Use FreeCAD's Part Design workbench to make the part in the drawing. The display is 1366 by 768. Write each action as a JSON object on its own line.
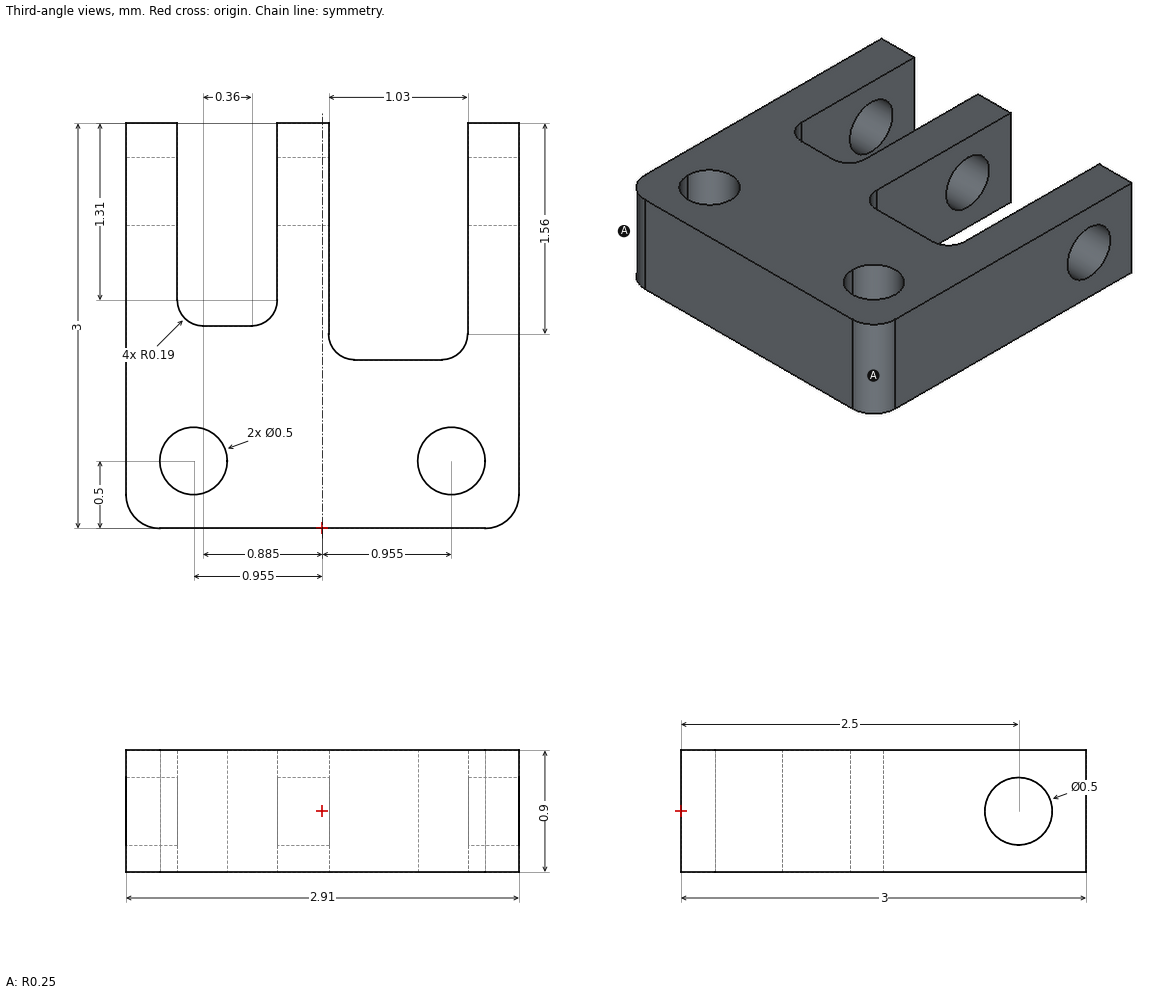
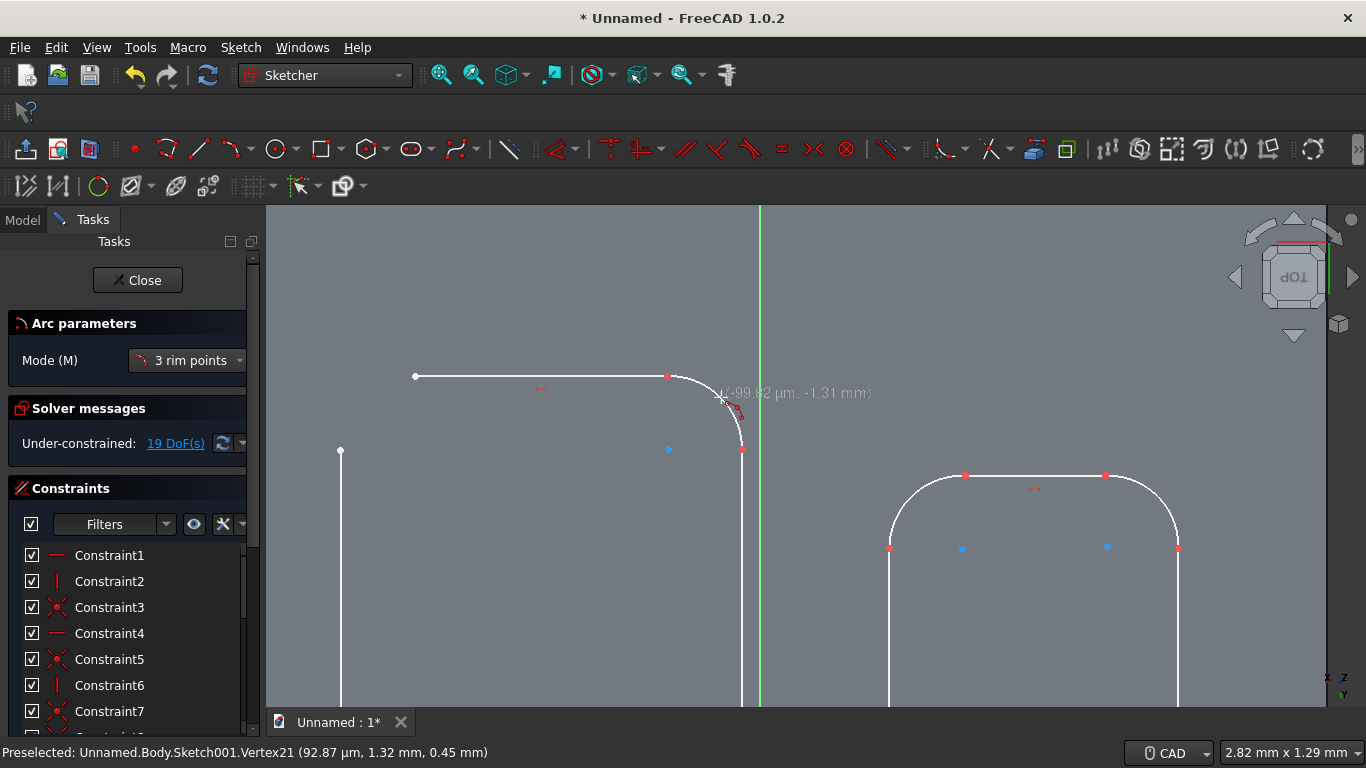
{"action": "left_click", "coordinate": [415, 376]}
{"action": "left_click", "coordinate": [341, 450]}
{"action": "left_click", "coordinate": [363, 397]}
{"action": "key", "text": "Escape"}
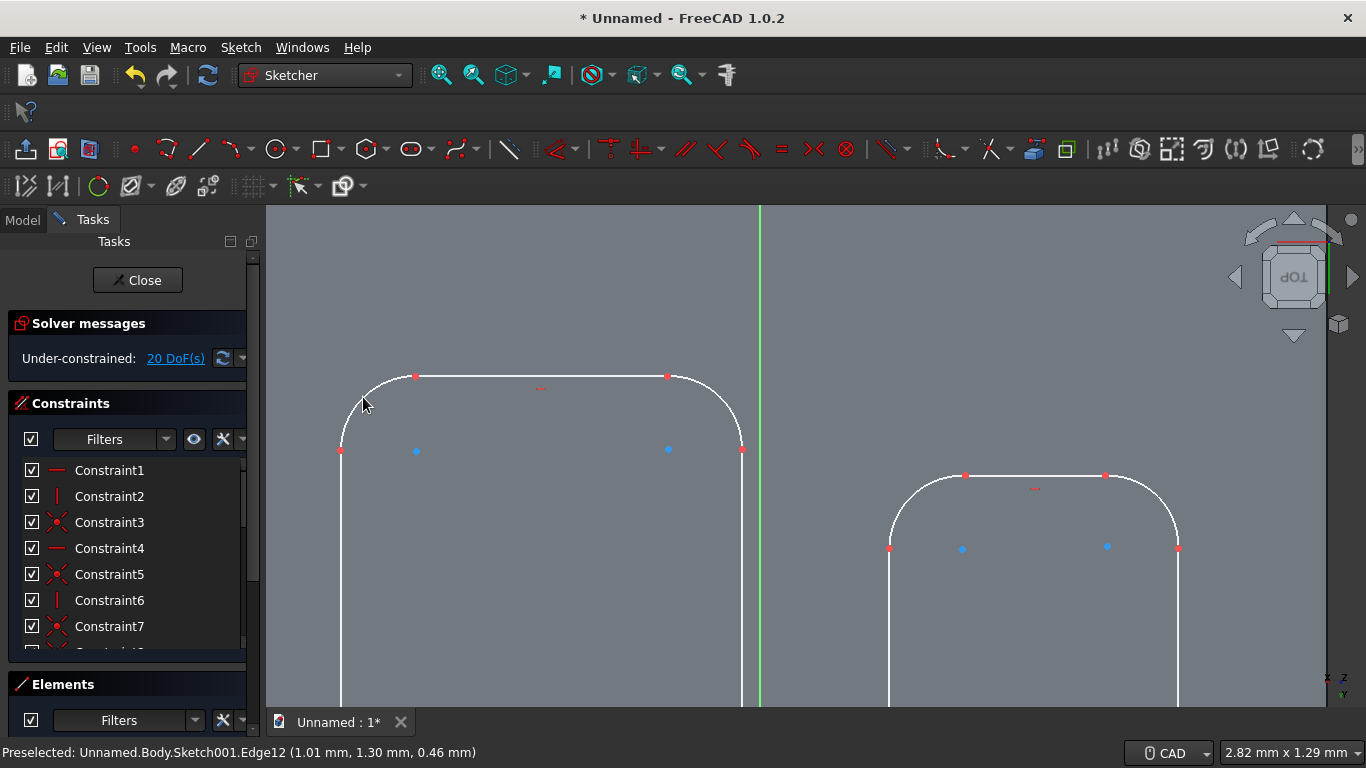
{"action": "left_click", "coordinate": [1063, 476]}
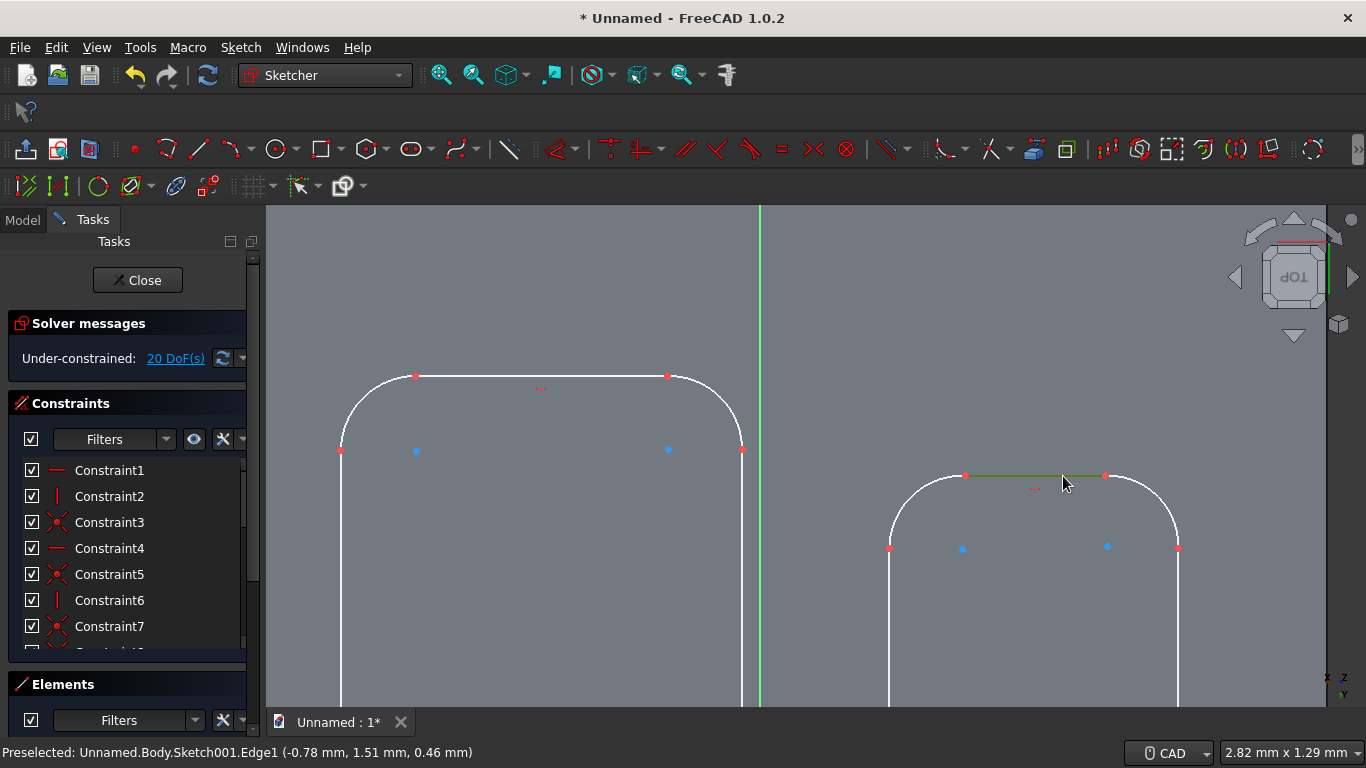
{"action": "left_click", "coordinate": [931, 483]}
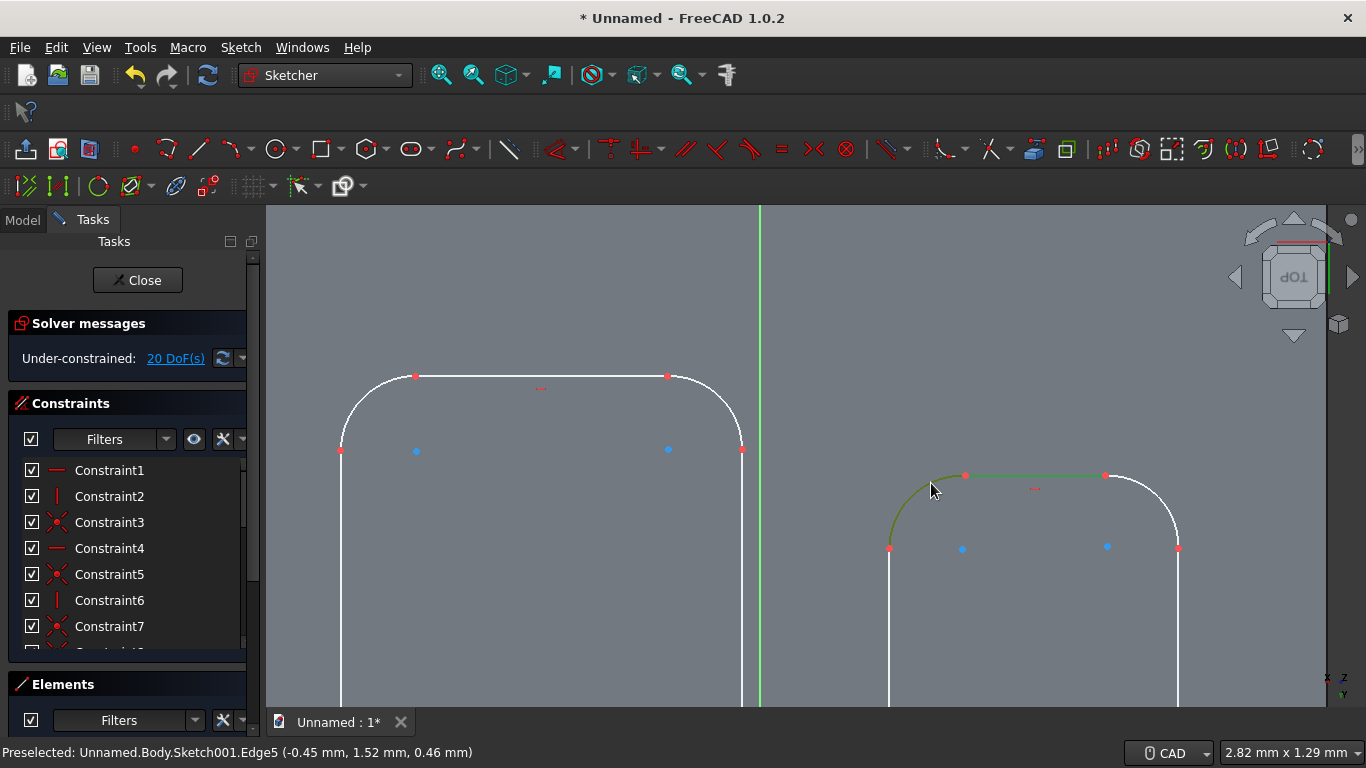
{"action": "key", "text": "t"}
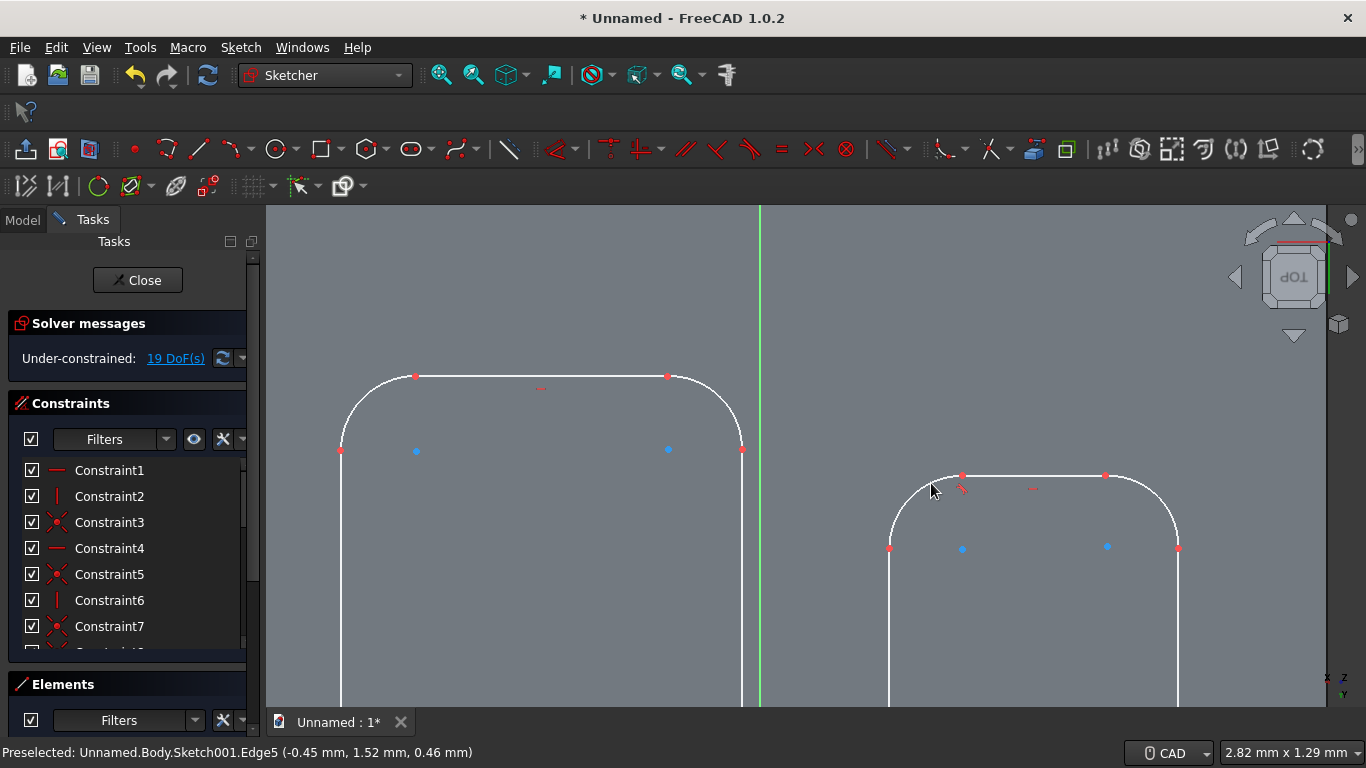
{"action": "left_click", "coordinate": [1062, 476]}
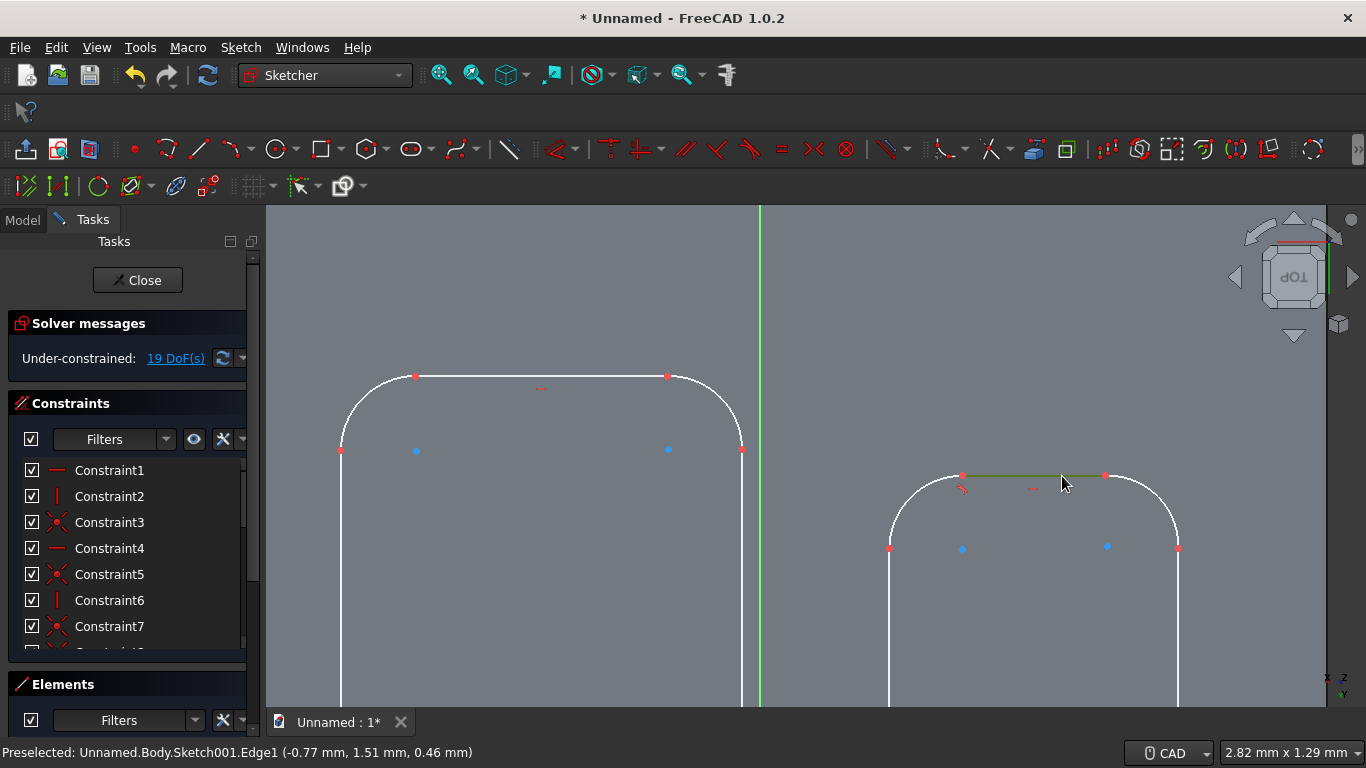
{"action": "left_click", "coordinate": [1171, 515]}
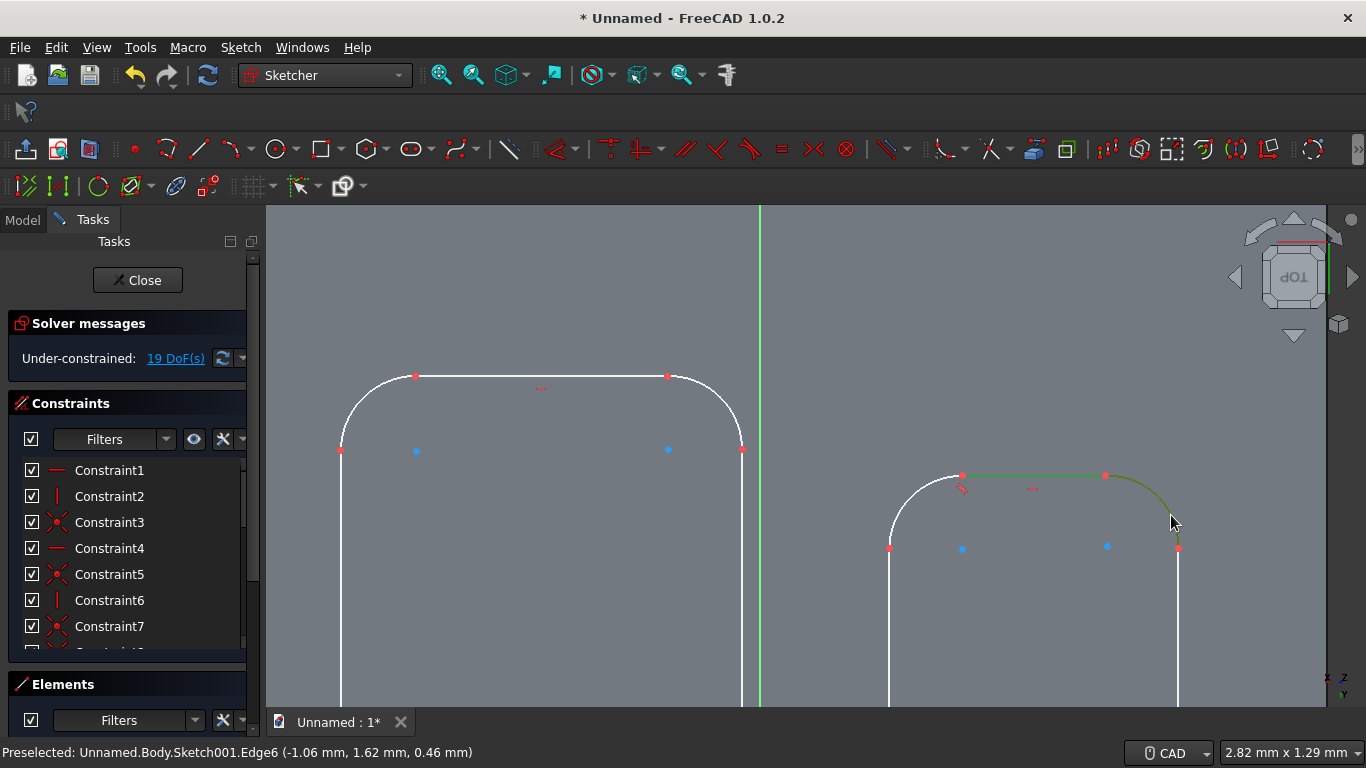
{"action": "key", "text": "t"}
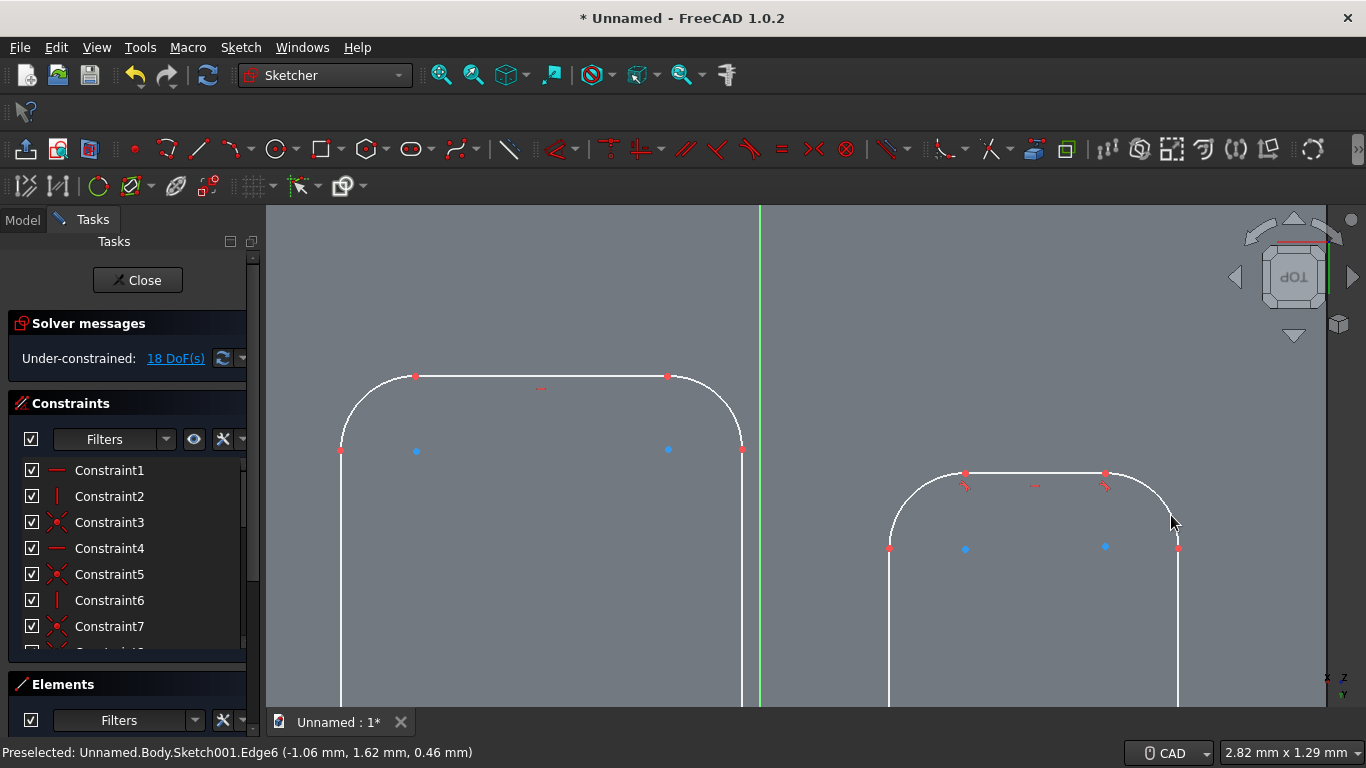
{"action": "left_click", "coordinate": [889, 651]}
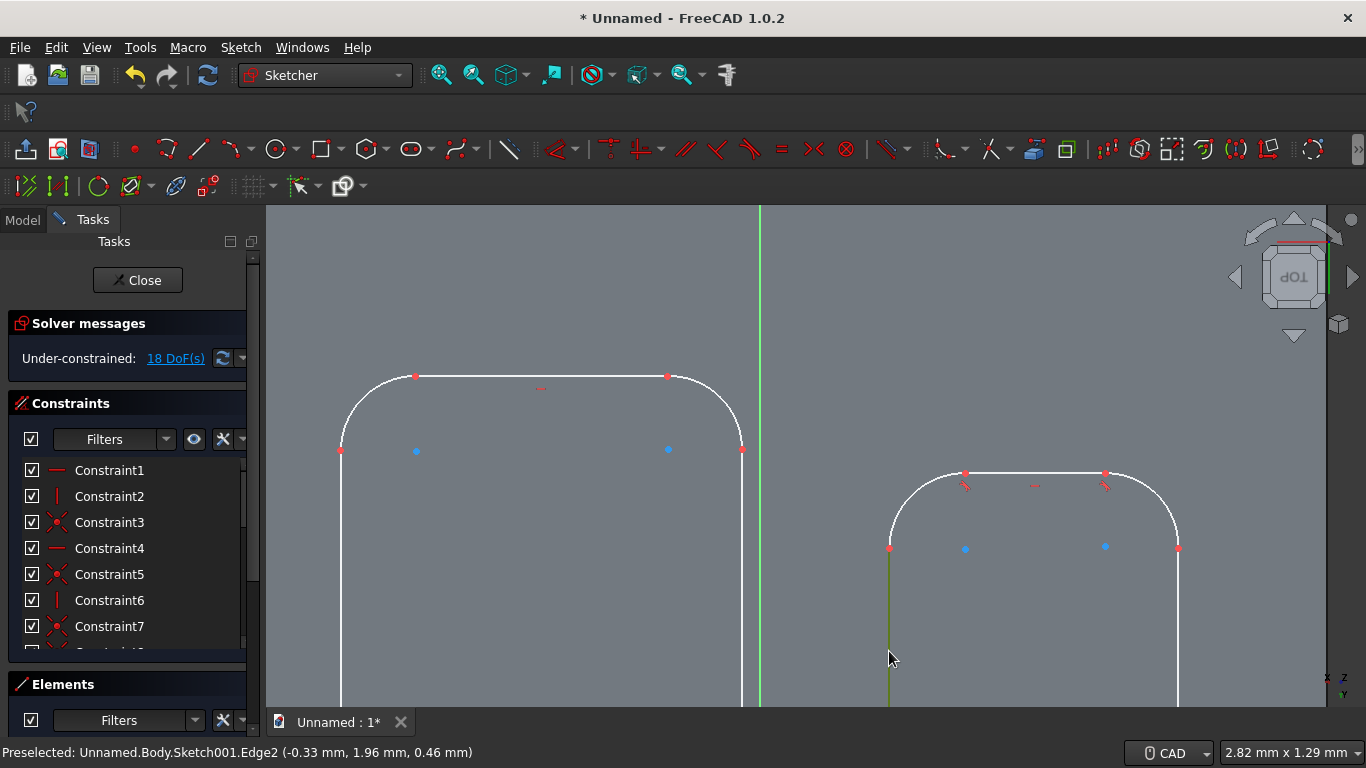
{"action": "left_click", "coordinate": [931, 481]}